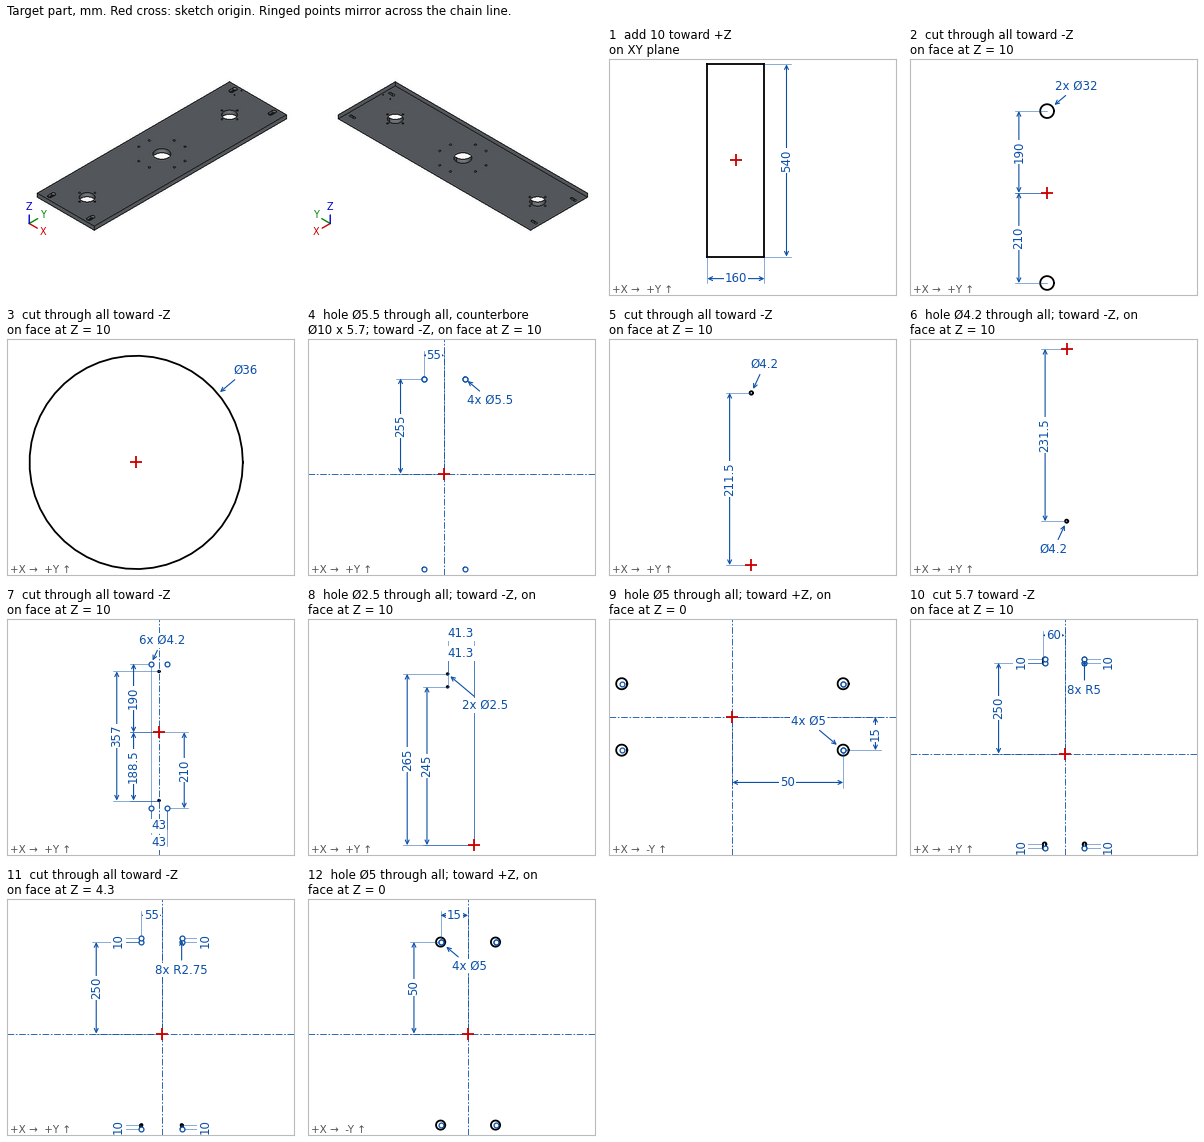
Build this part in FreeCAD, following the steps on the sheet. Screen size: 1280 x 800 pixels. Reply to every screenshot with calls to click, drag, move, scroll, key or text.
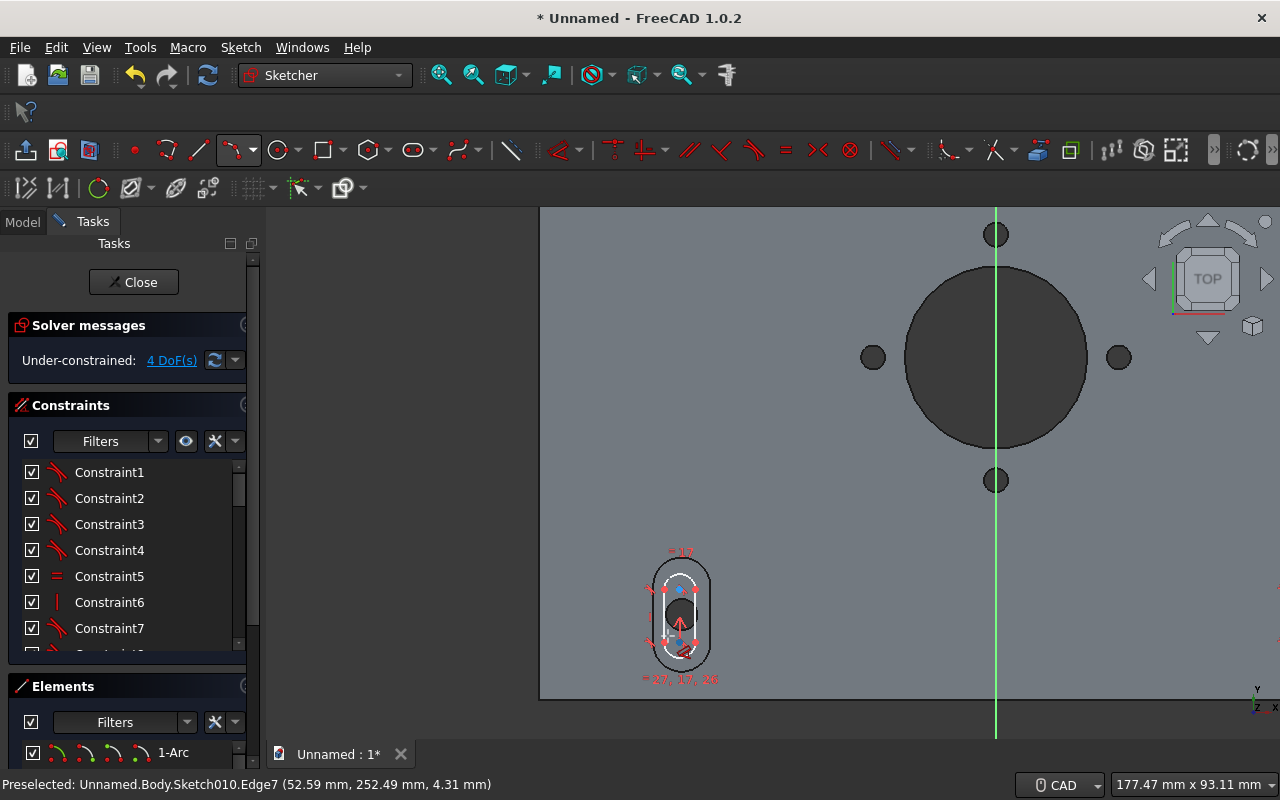
click(664, 626)
click(630, 616)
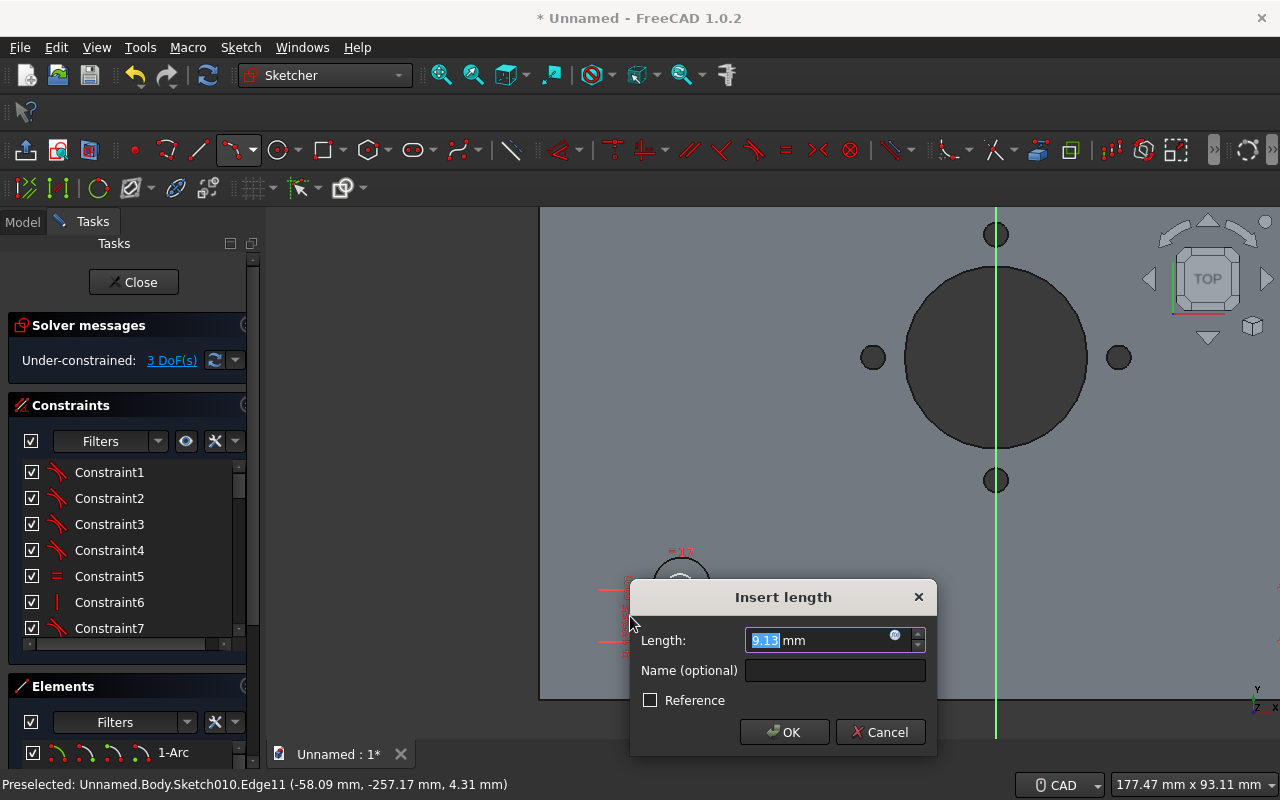
text(10)
key(Return)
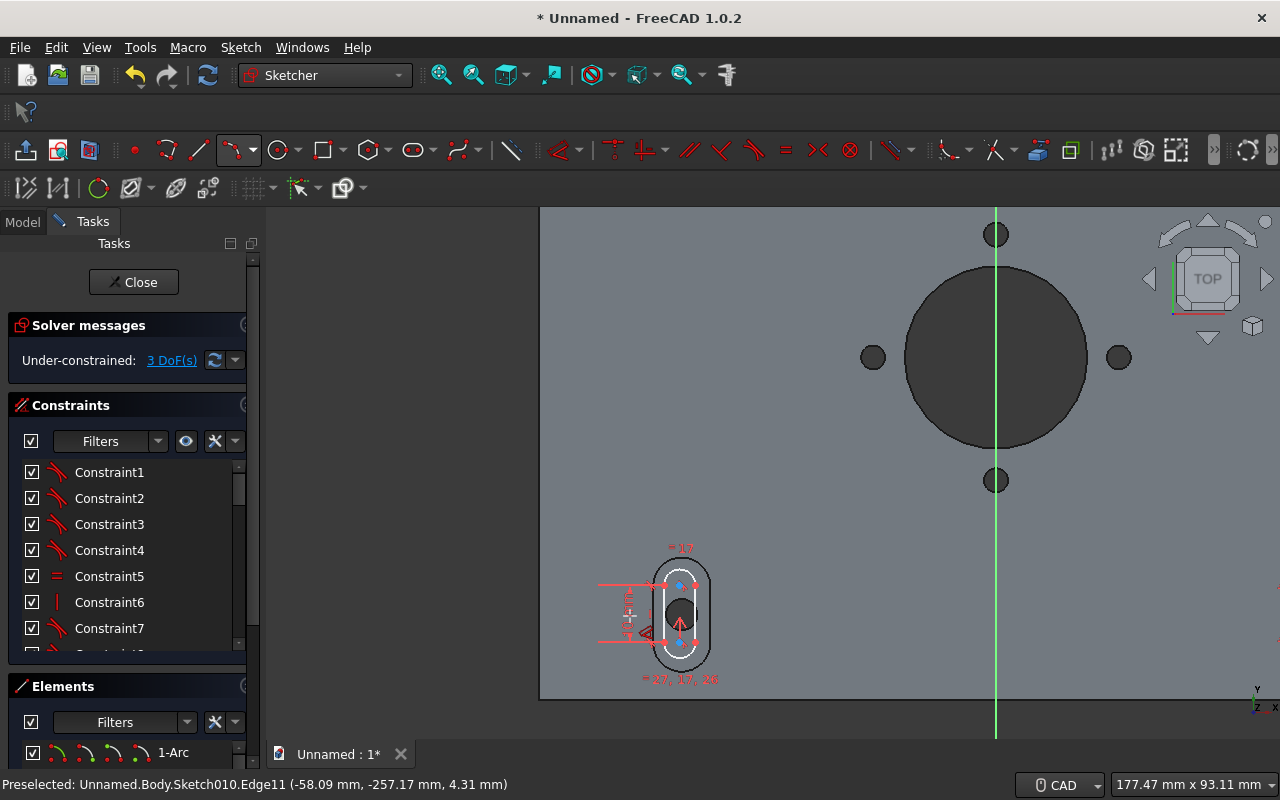
scroll(668, 637, down, 11)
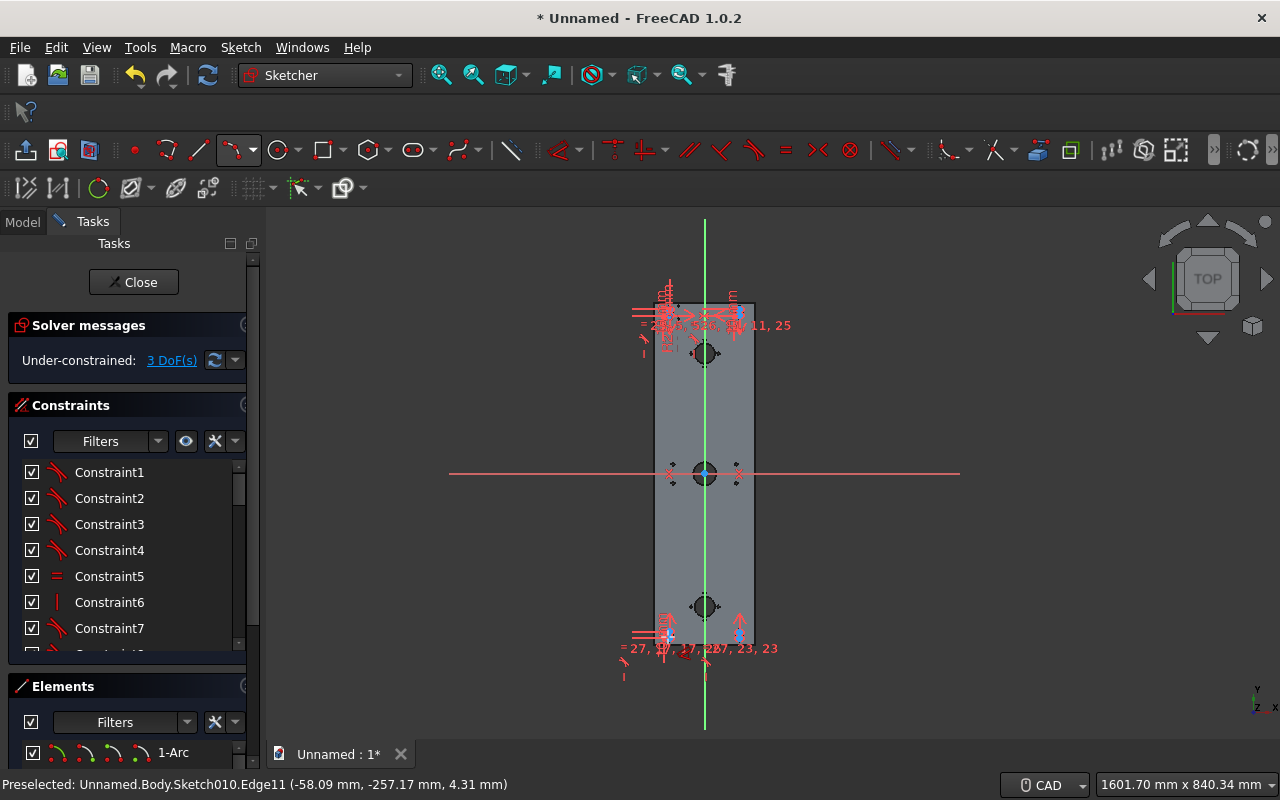
scroll(738, 637, up, 11)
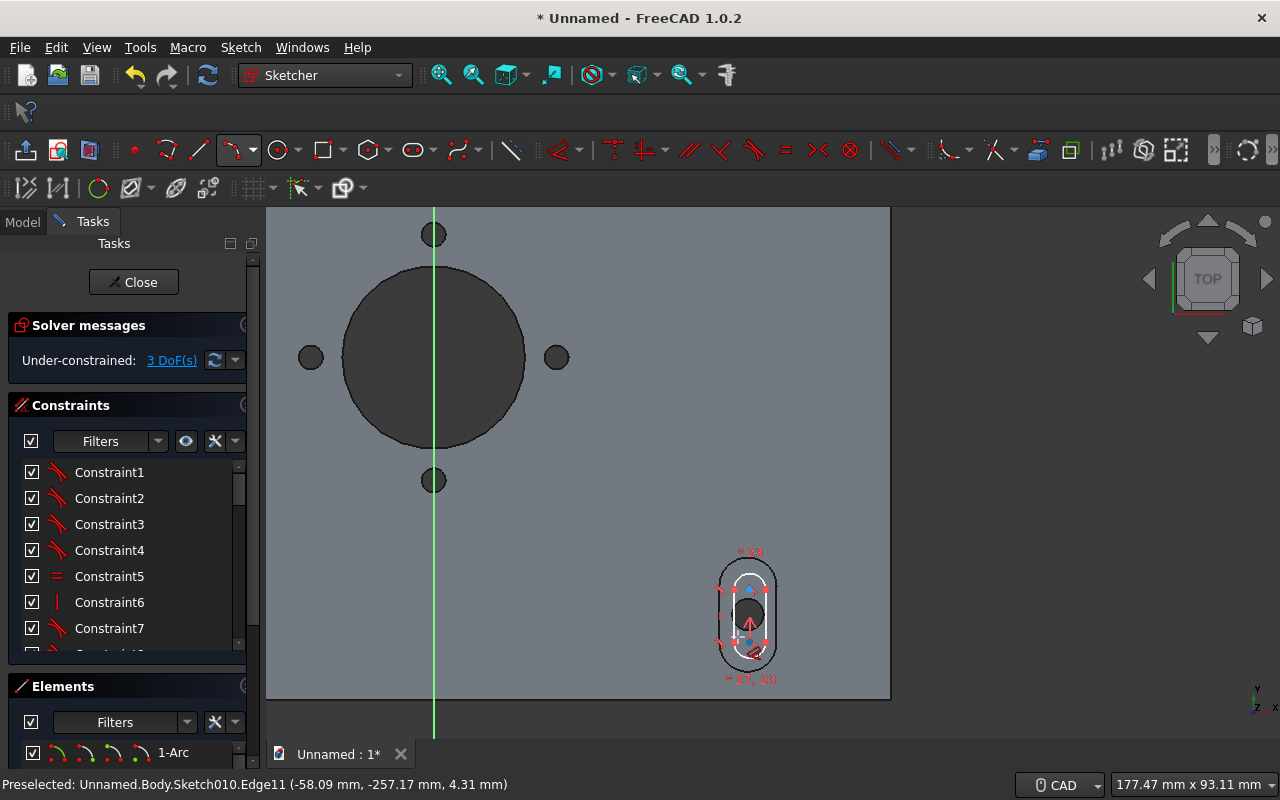
click(734, 626)
click(700, 616)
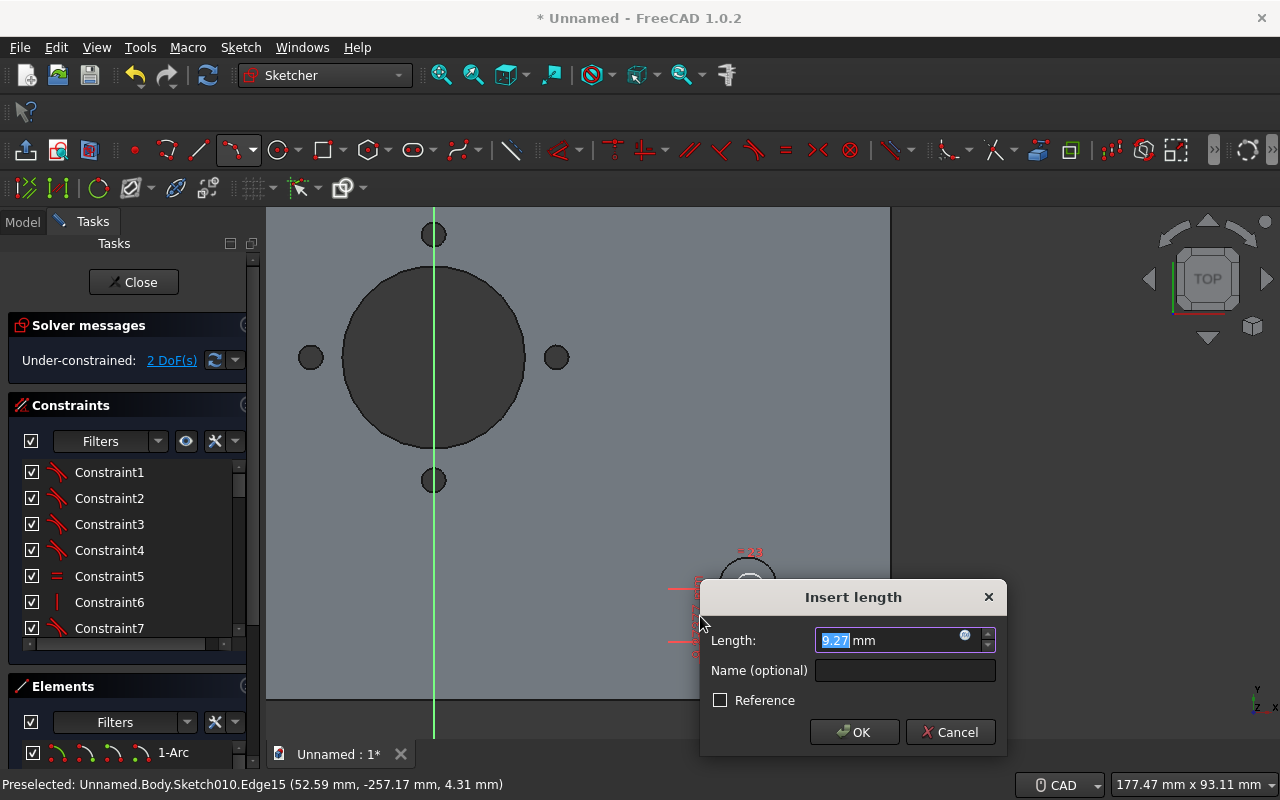
text(10)
key(Return)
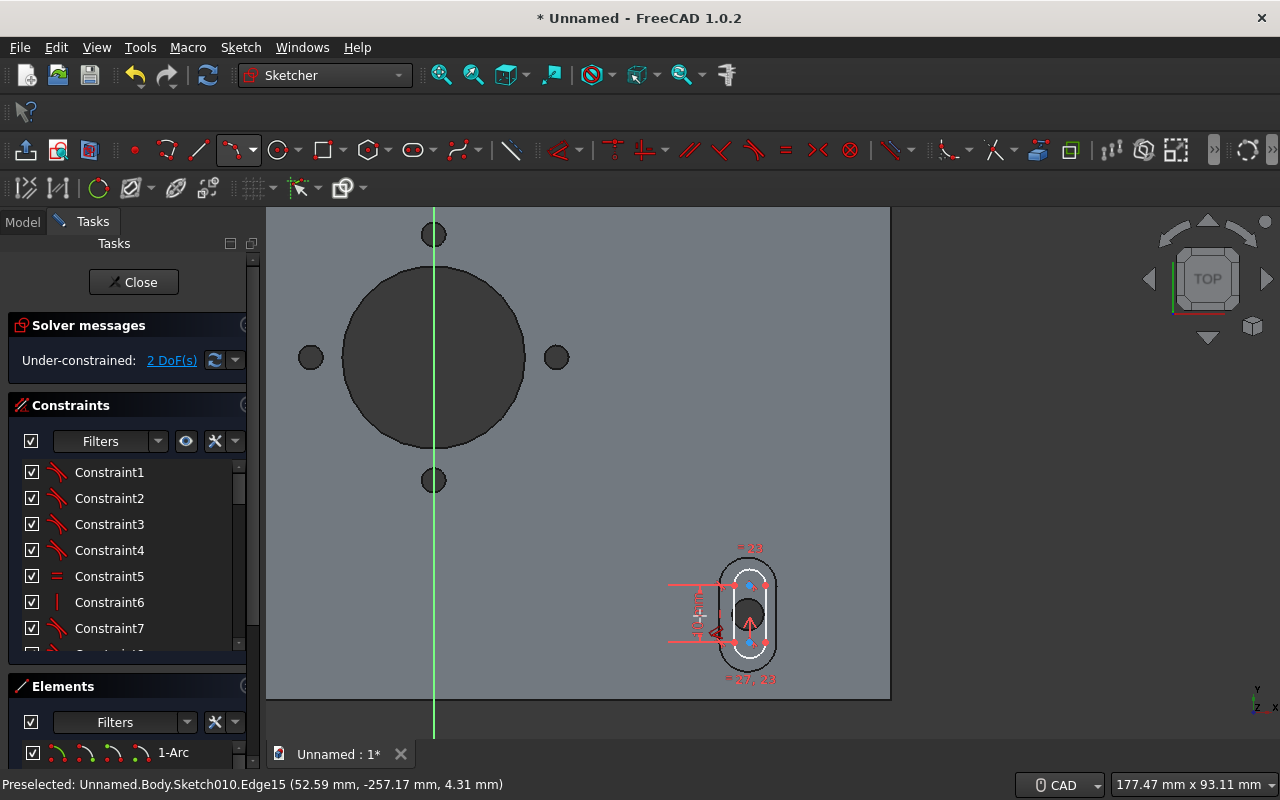
scroll(738, 637, down, 11)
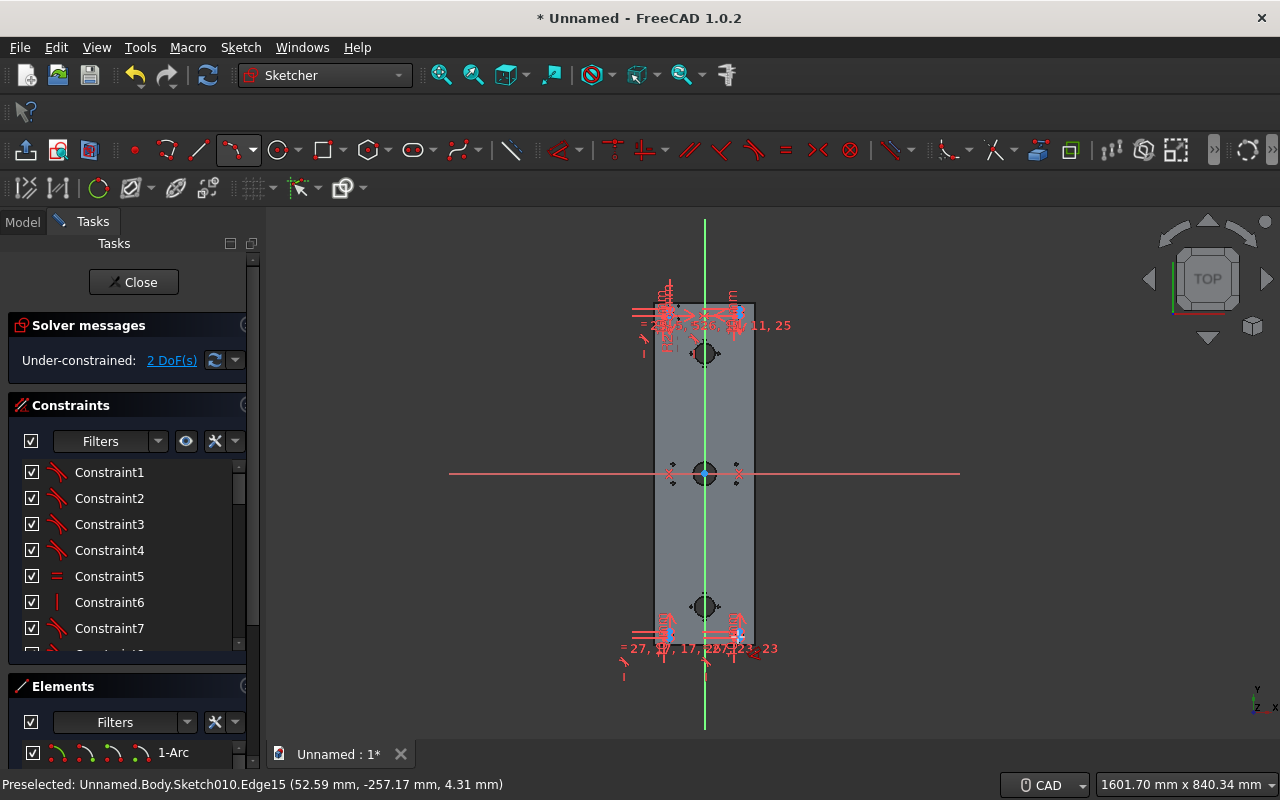
scroll(670, 316, up, 10)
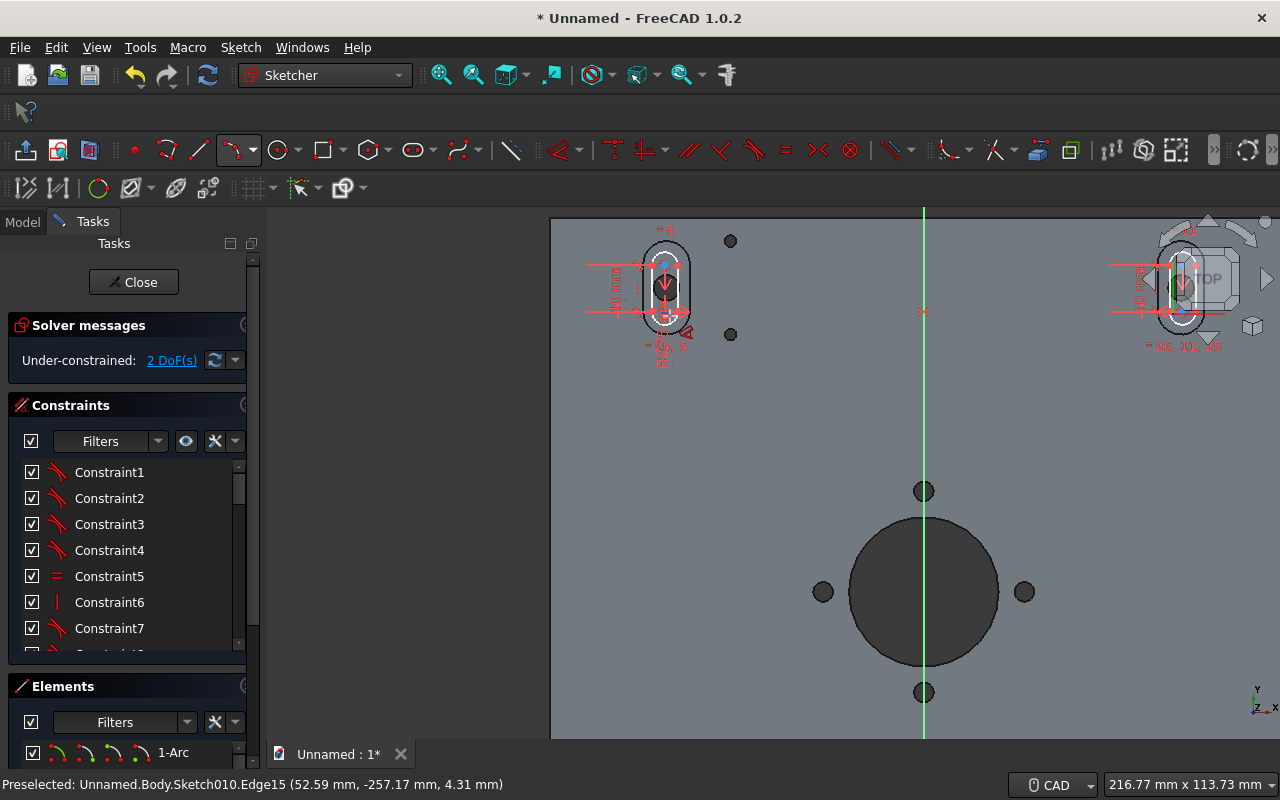
click(665, 312)
click(794, 278)